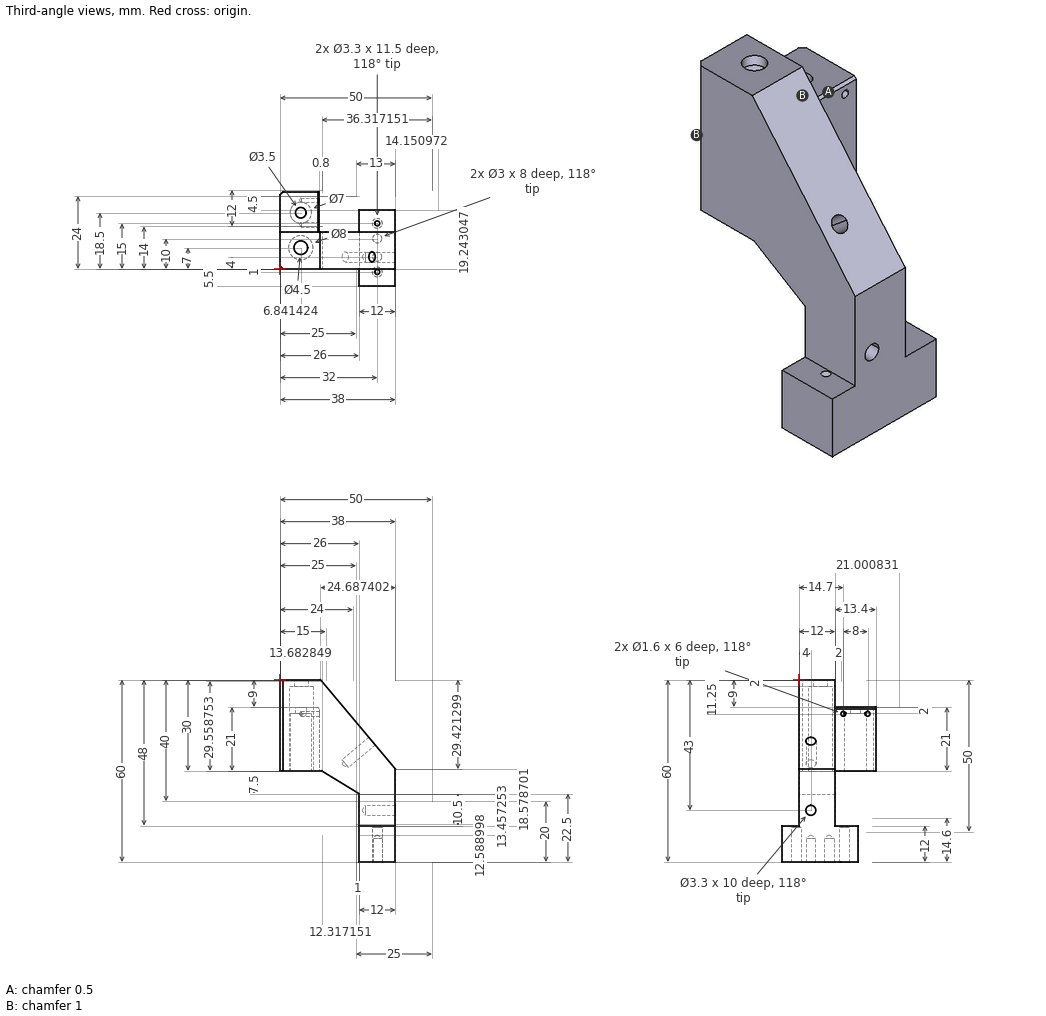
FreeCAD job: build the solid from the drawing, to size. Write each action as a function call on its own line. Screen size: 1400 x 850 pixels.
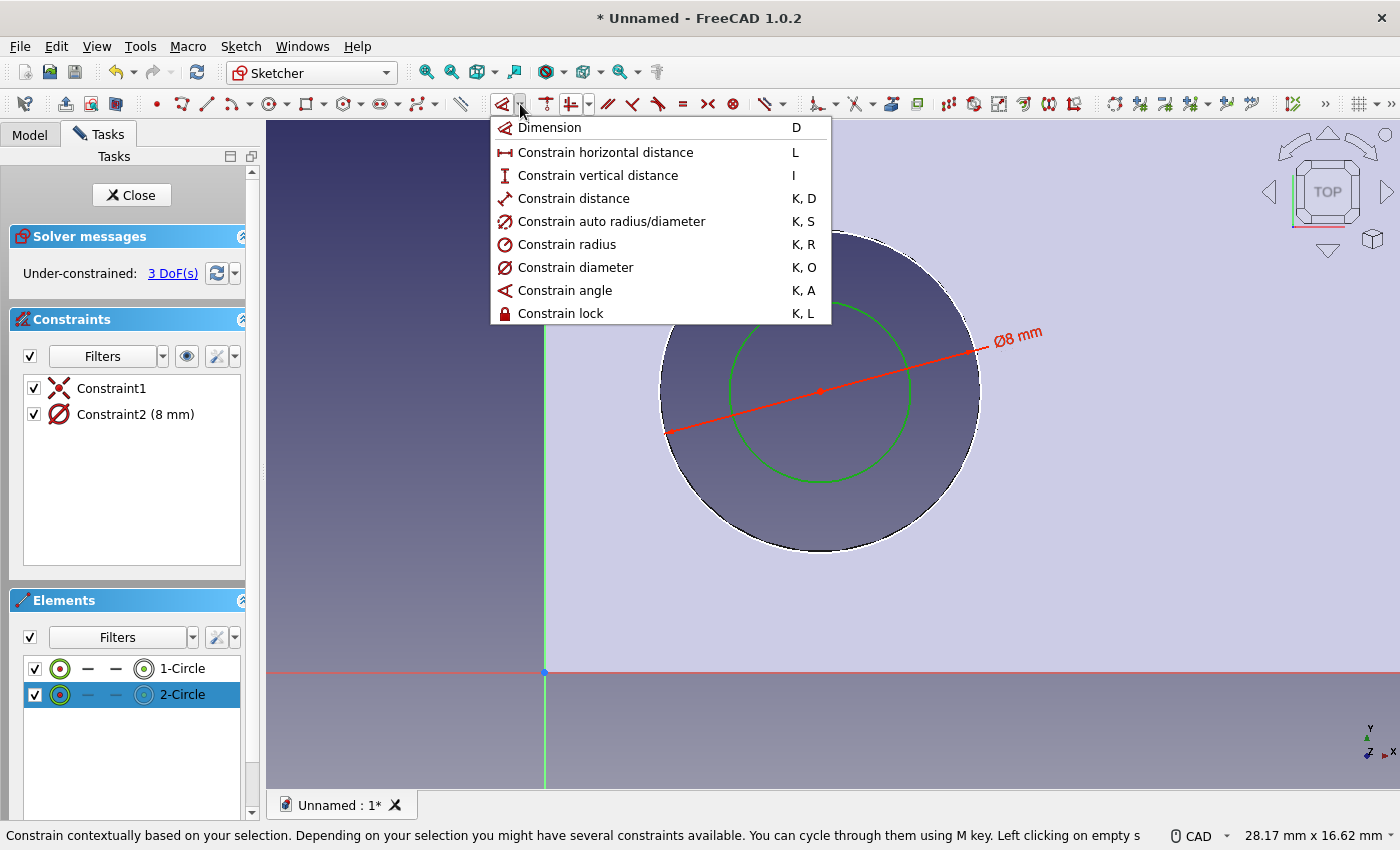
click(661, 268)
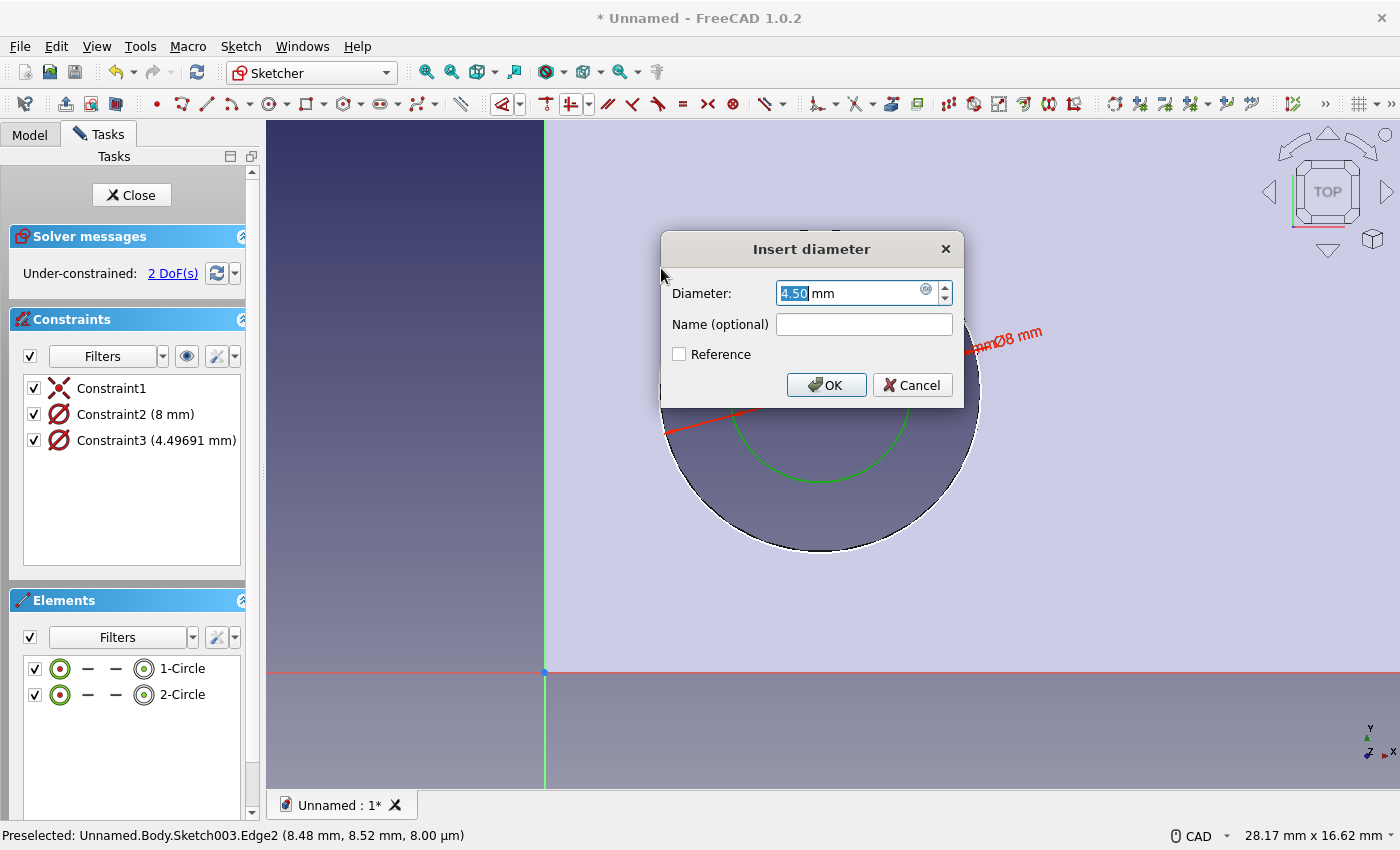
text(4.5)
key(Return)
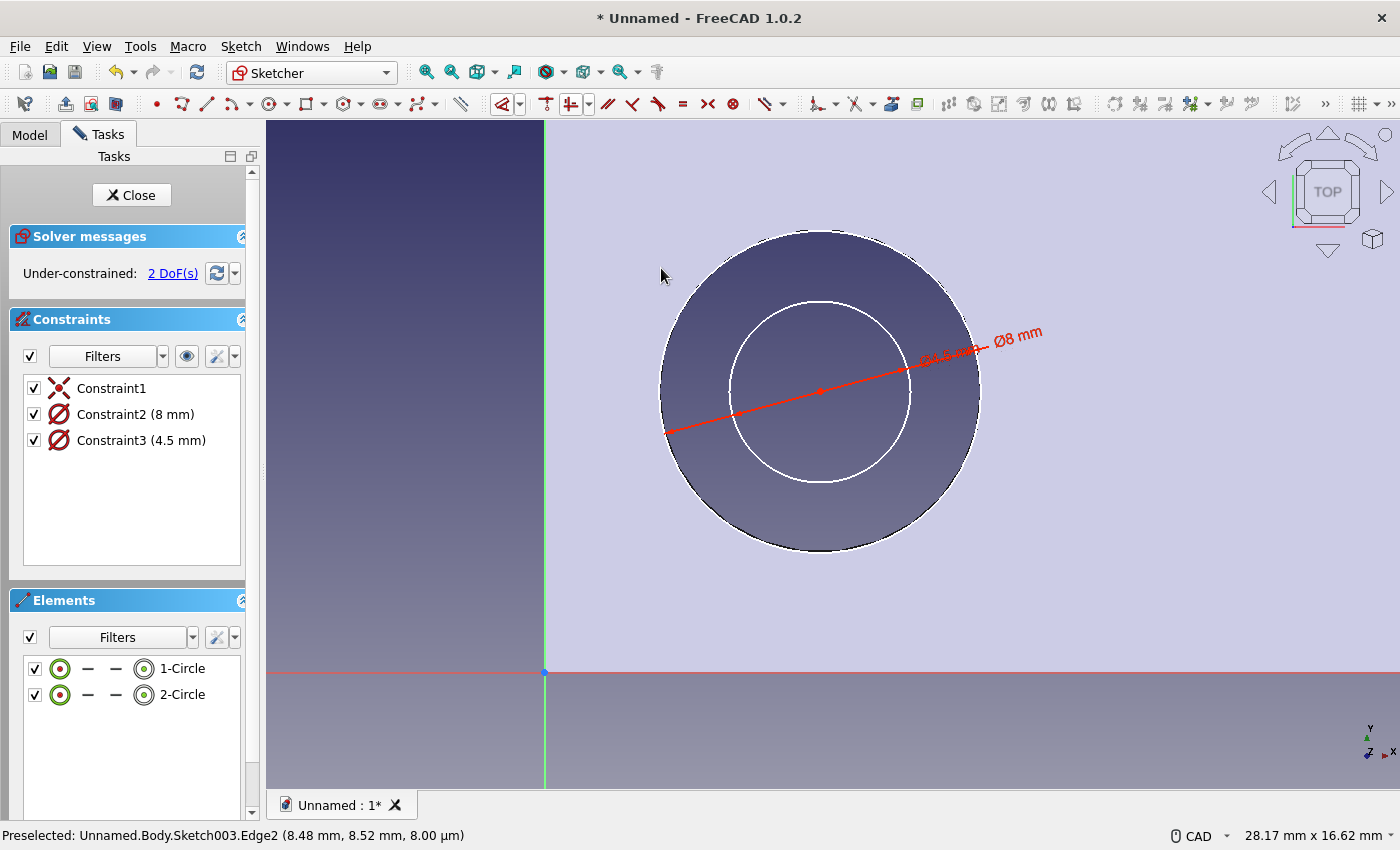
click(820, 392)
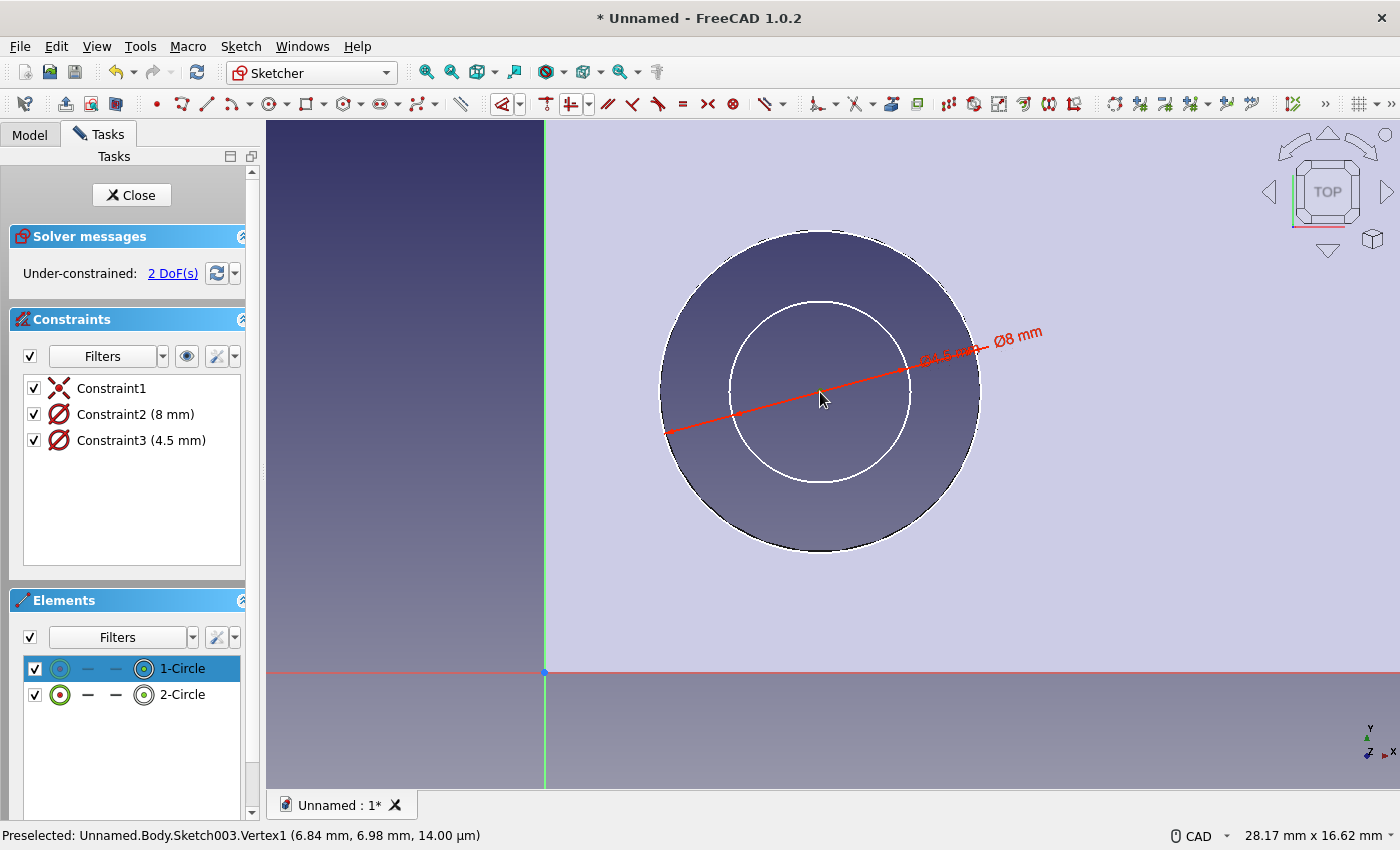
key(i)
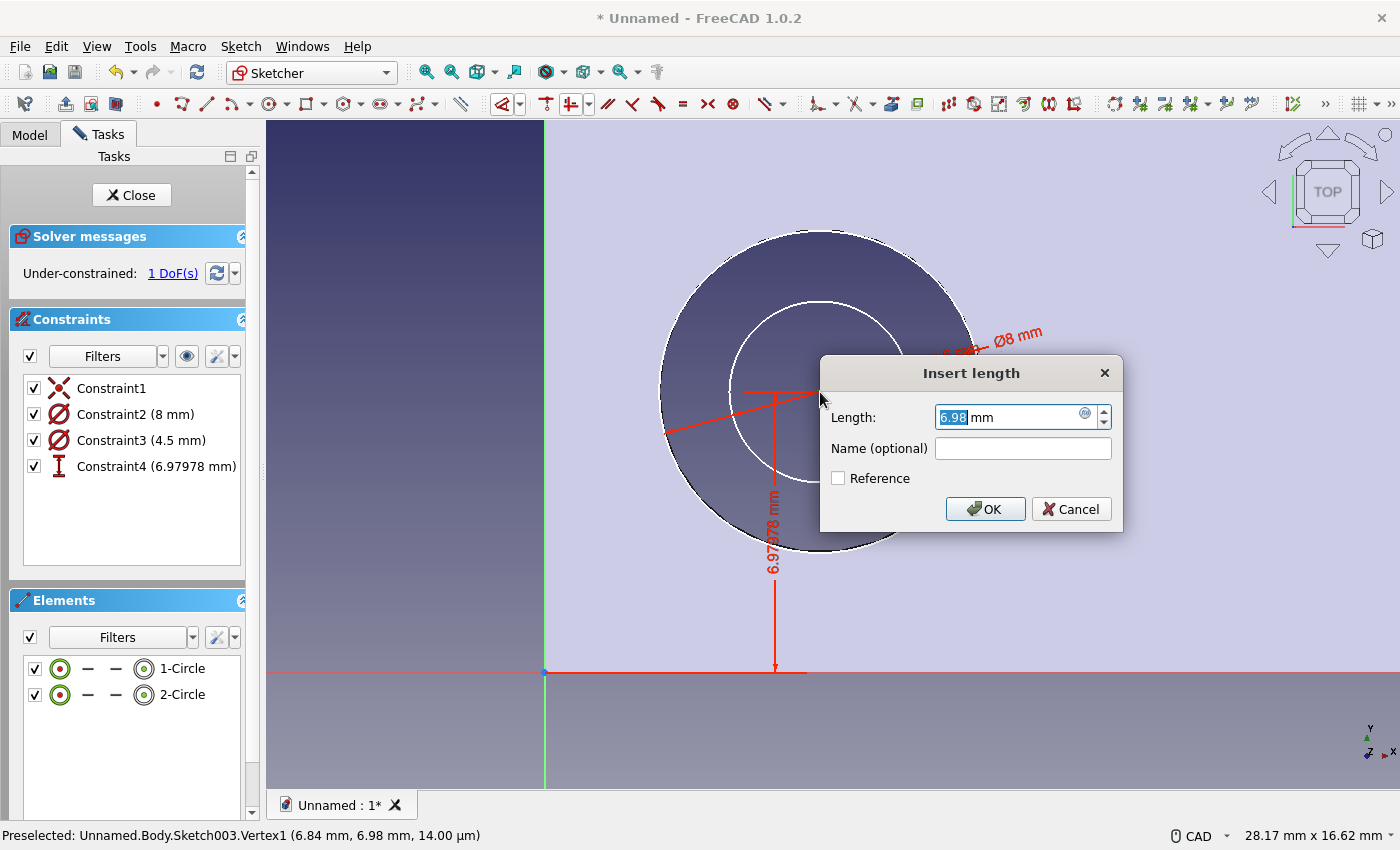
text(7)
key(Return)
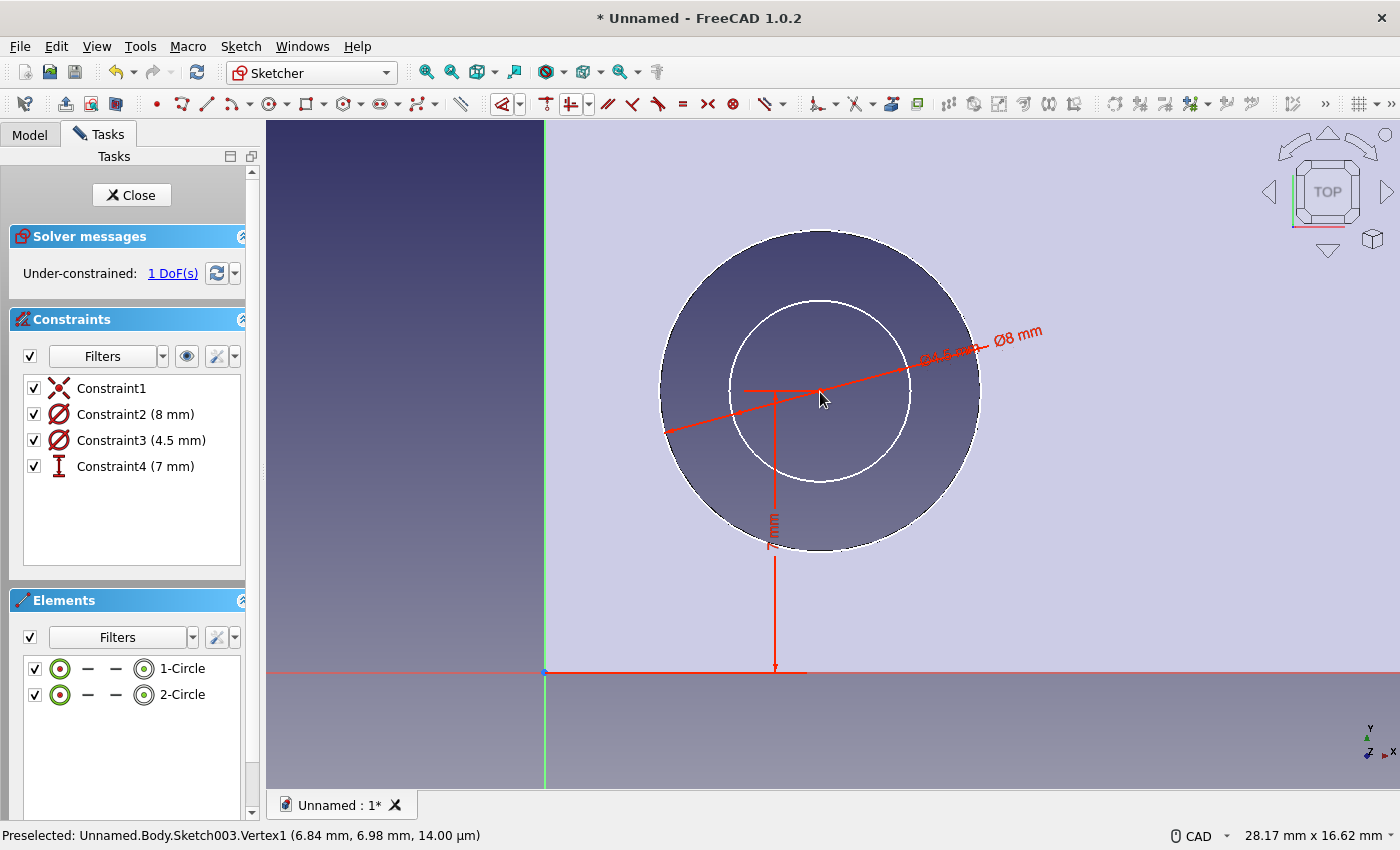
click(820, 391)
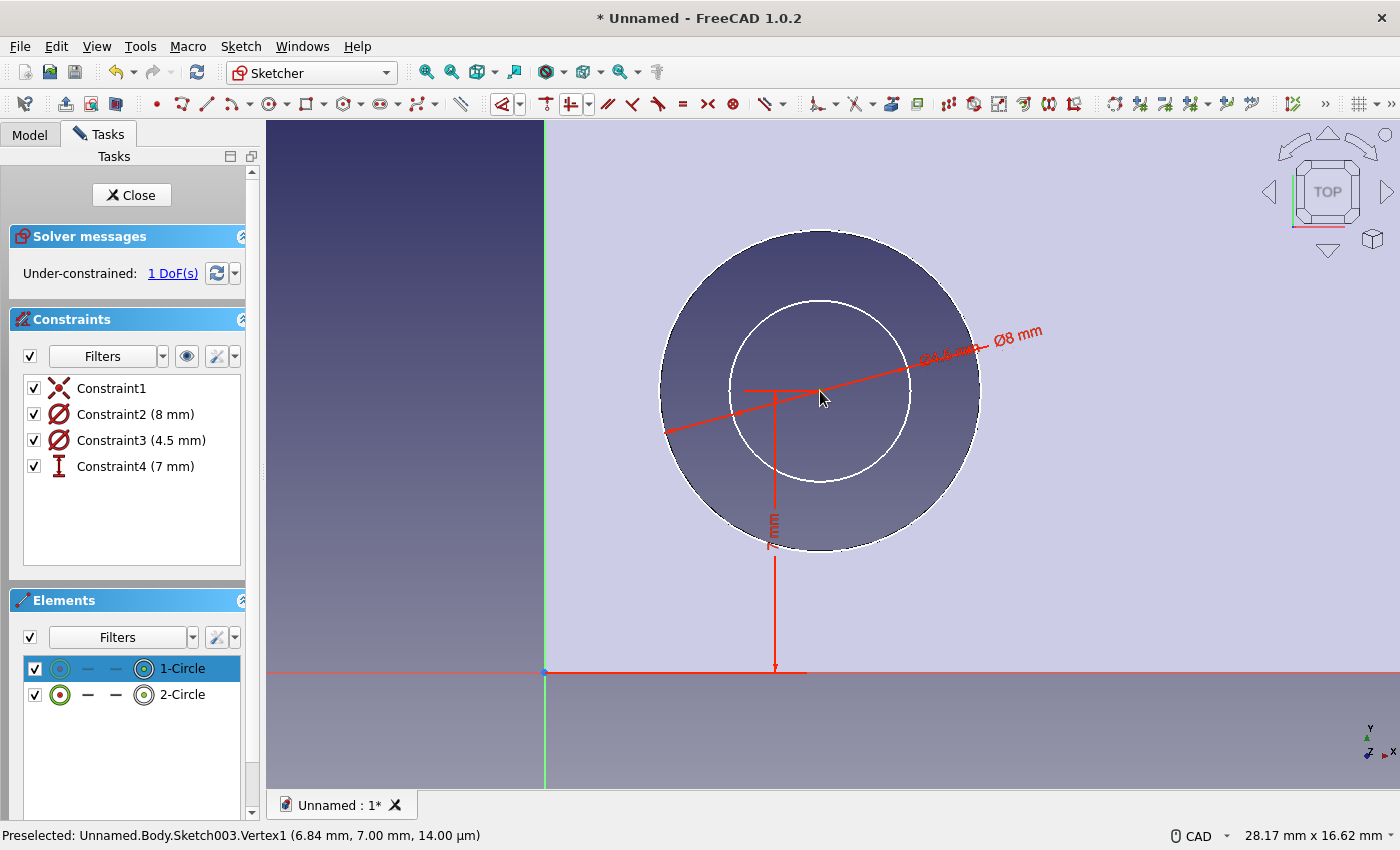
key(l)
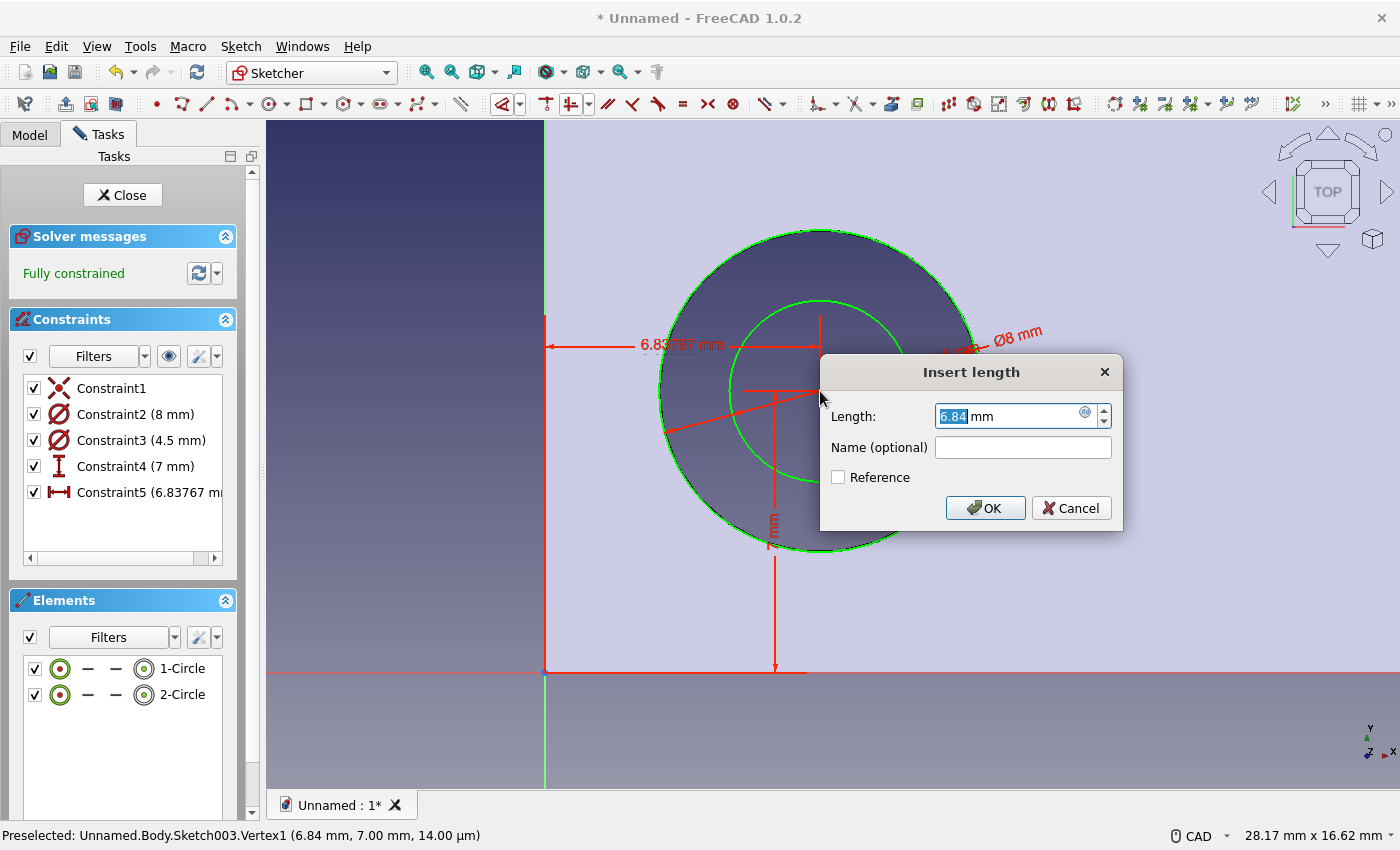
text(6.841424)
key(Return)